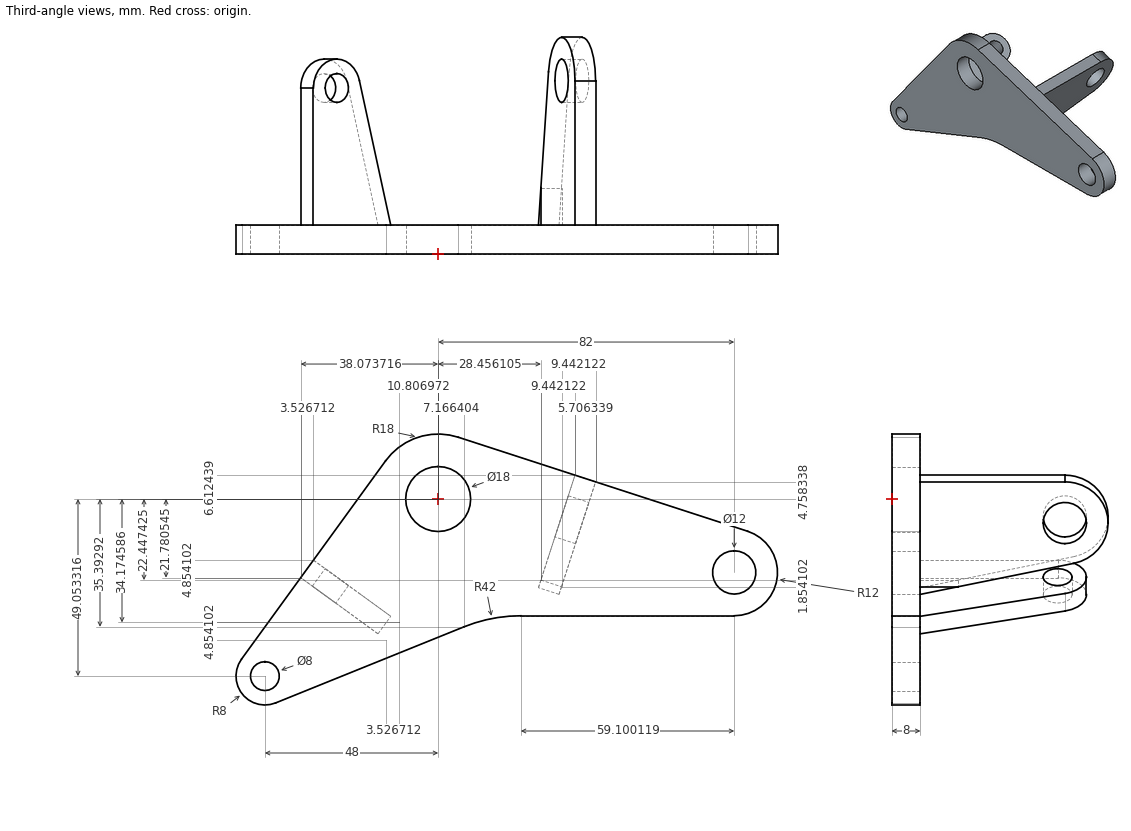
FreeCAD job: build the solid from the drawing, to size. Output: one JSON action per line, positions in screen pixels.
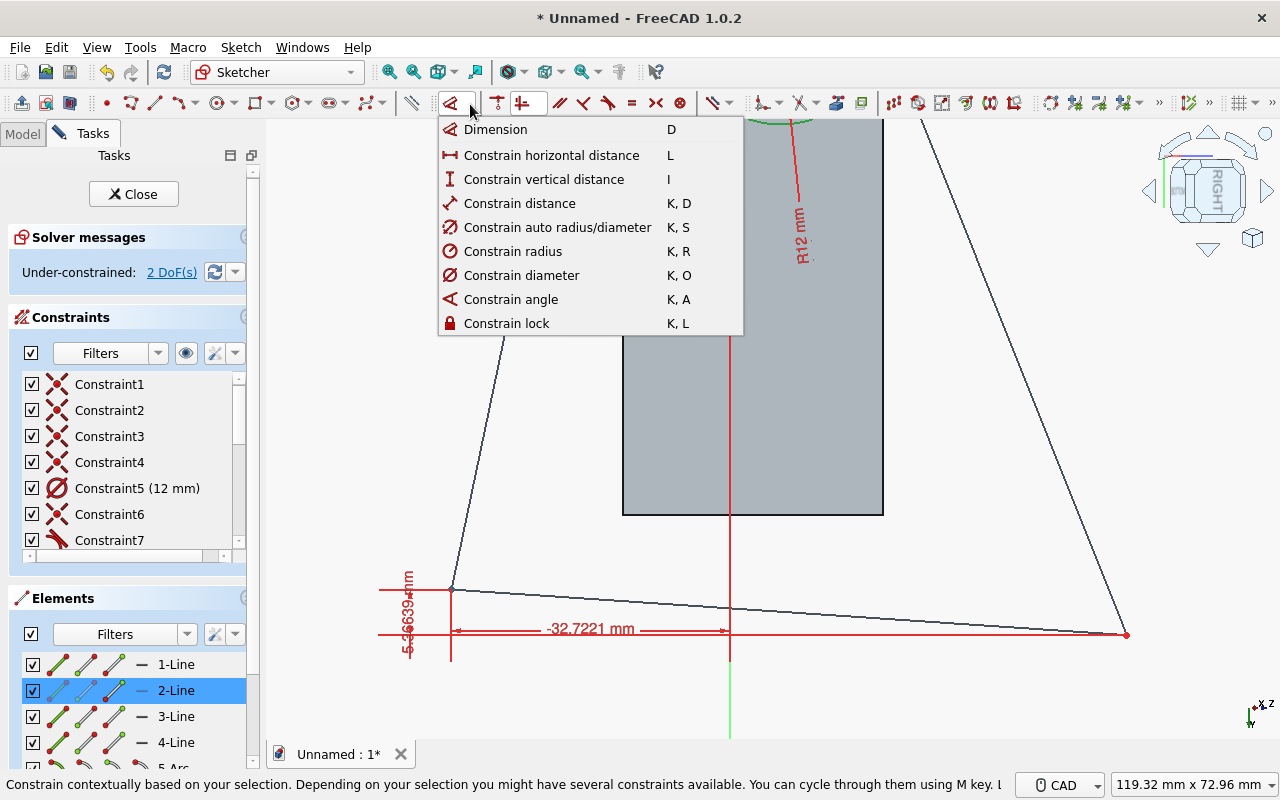
{"action": "left_click", "coordinate": [591, 179]}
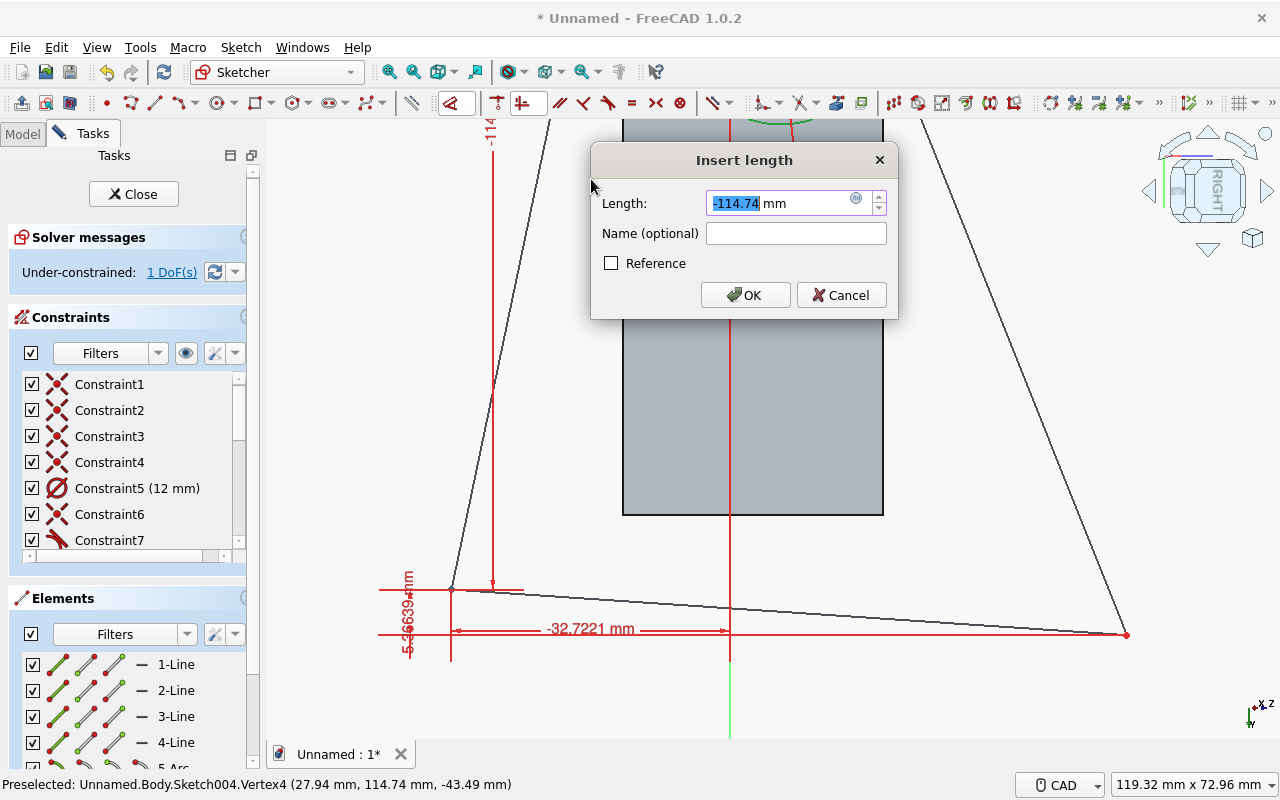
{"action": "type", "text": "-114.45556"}
{"action": "key", "text": "Return"}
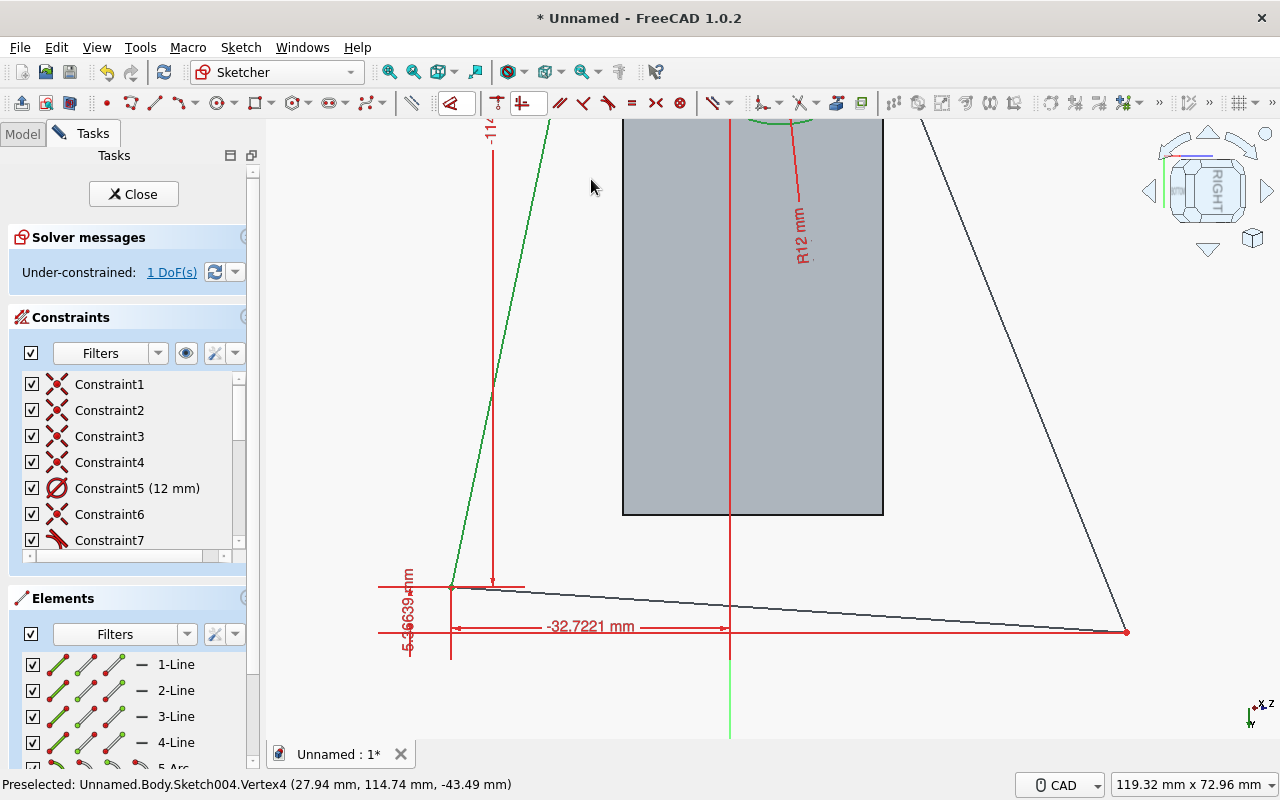
{"action": "scroll", "coordinate": [655, 607], "scroll_direction": "down", "scroll_amount": 5}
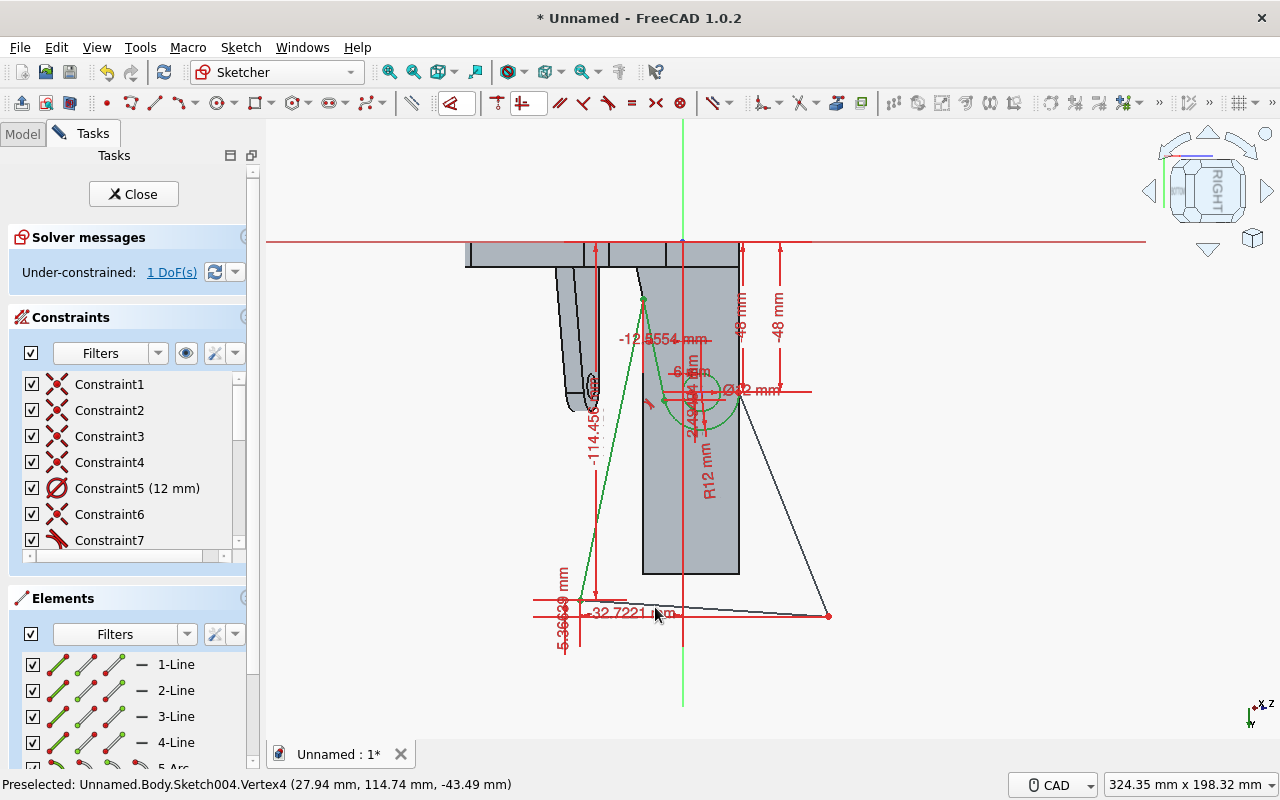
{"action": "left_click", "coordinate": [829, 617]}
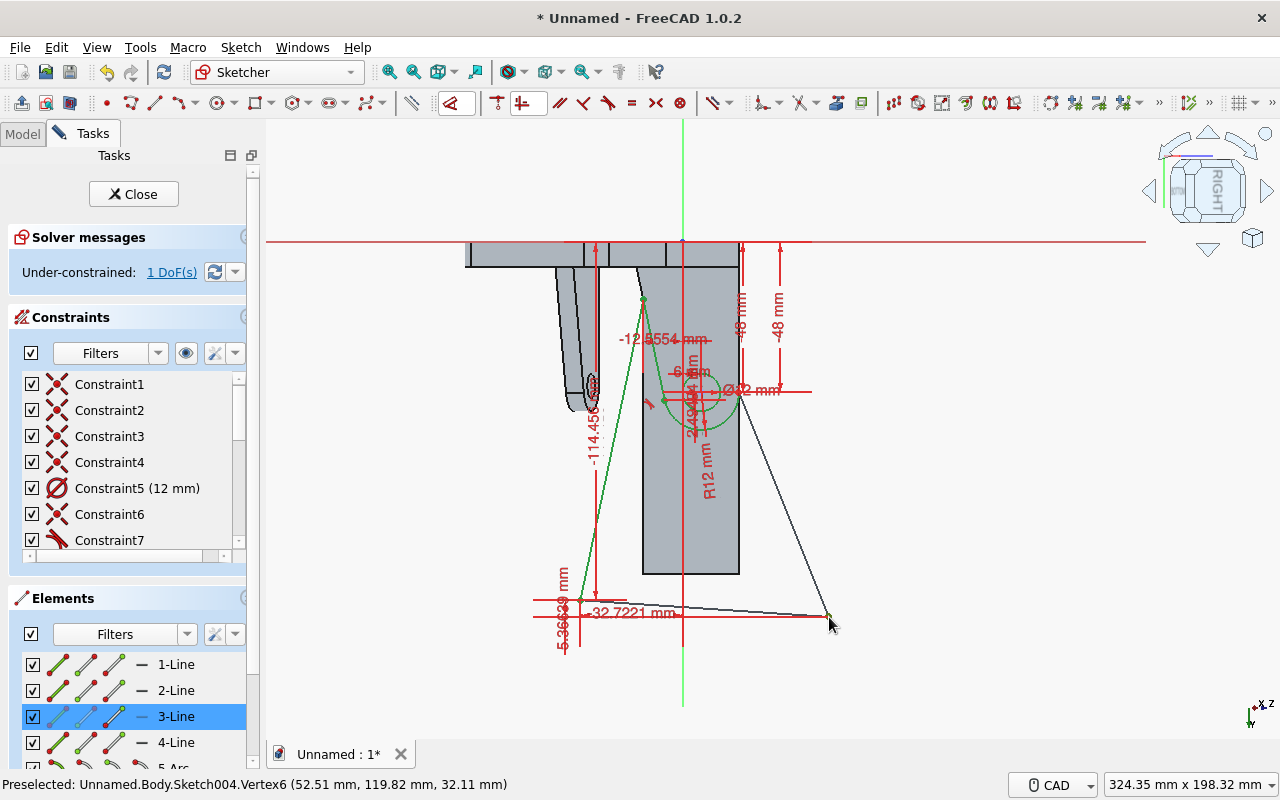
{"action": "key", "text": "l"}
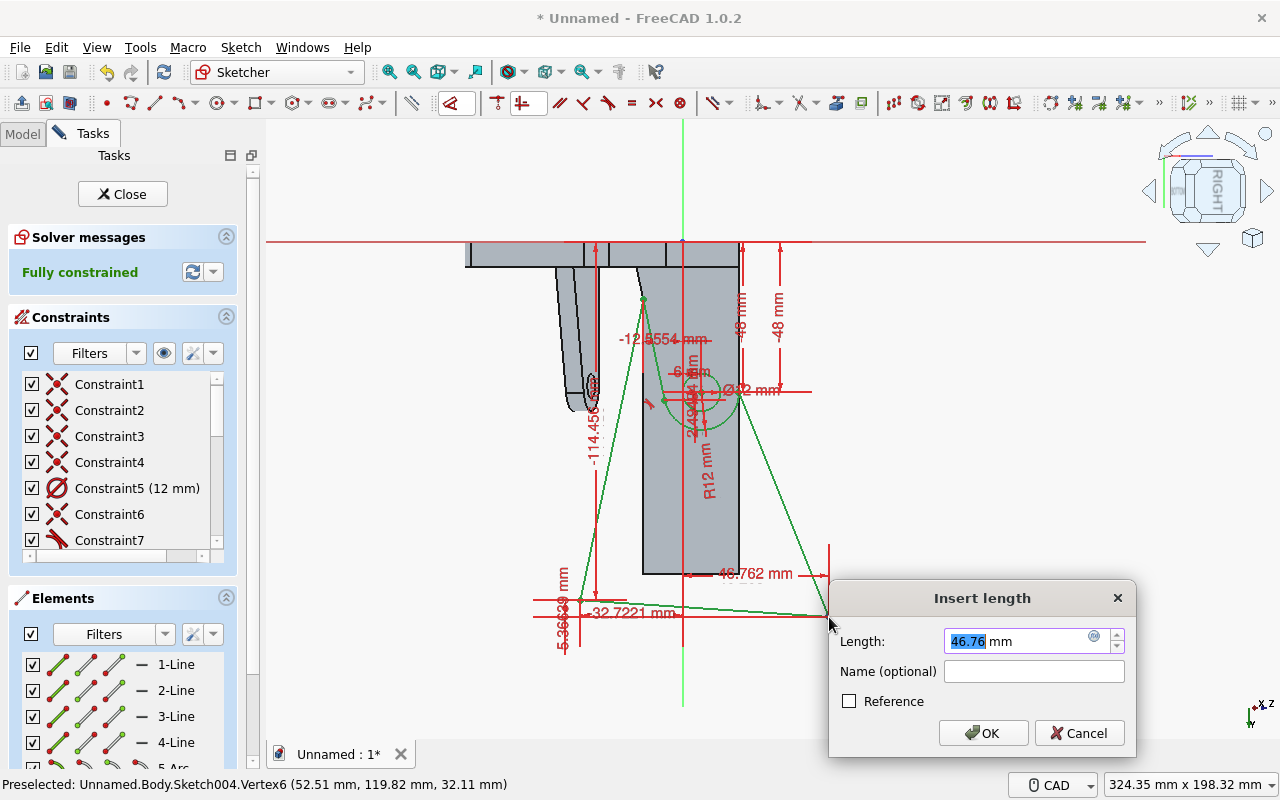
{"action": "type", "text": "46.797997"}
{"action": "key", "text": "Return"}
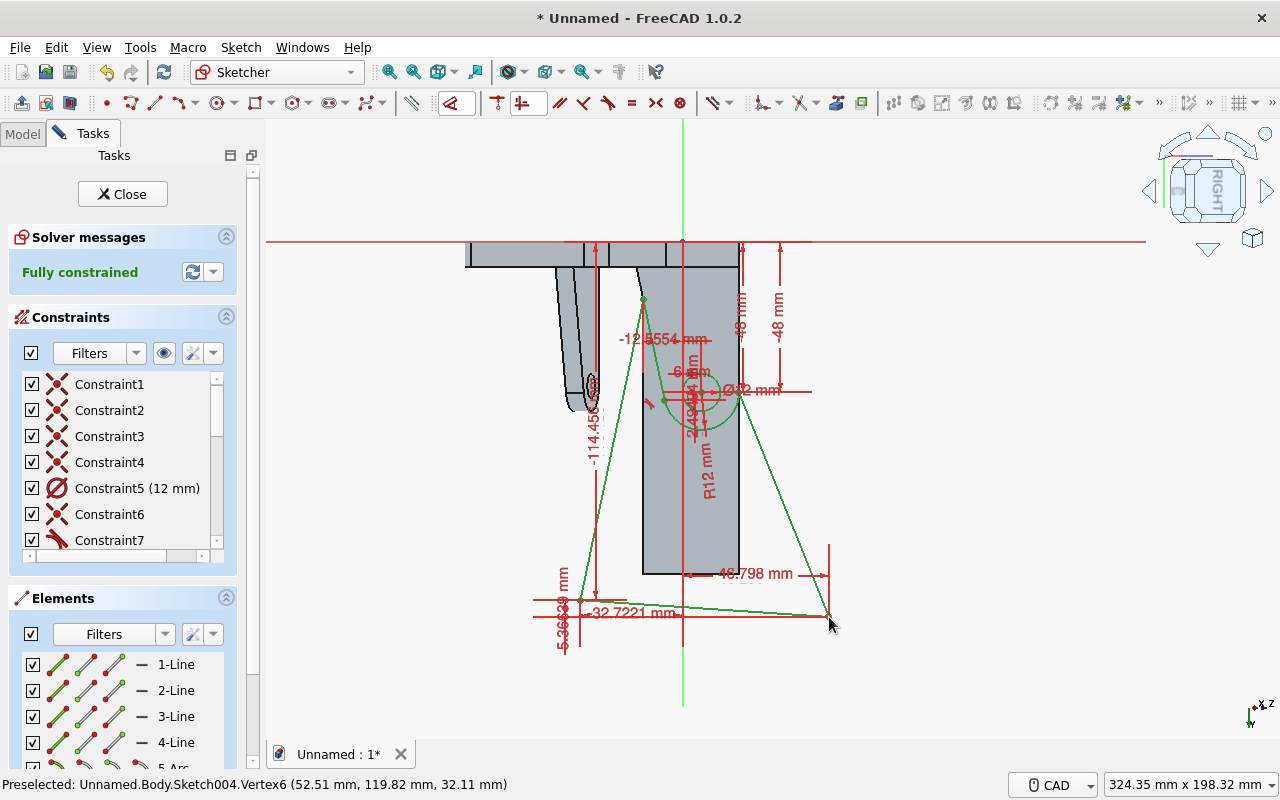
{"action": "left_click", "coordinate": [123, 194]}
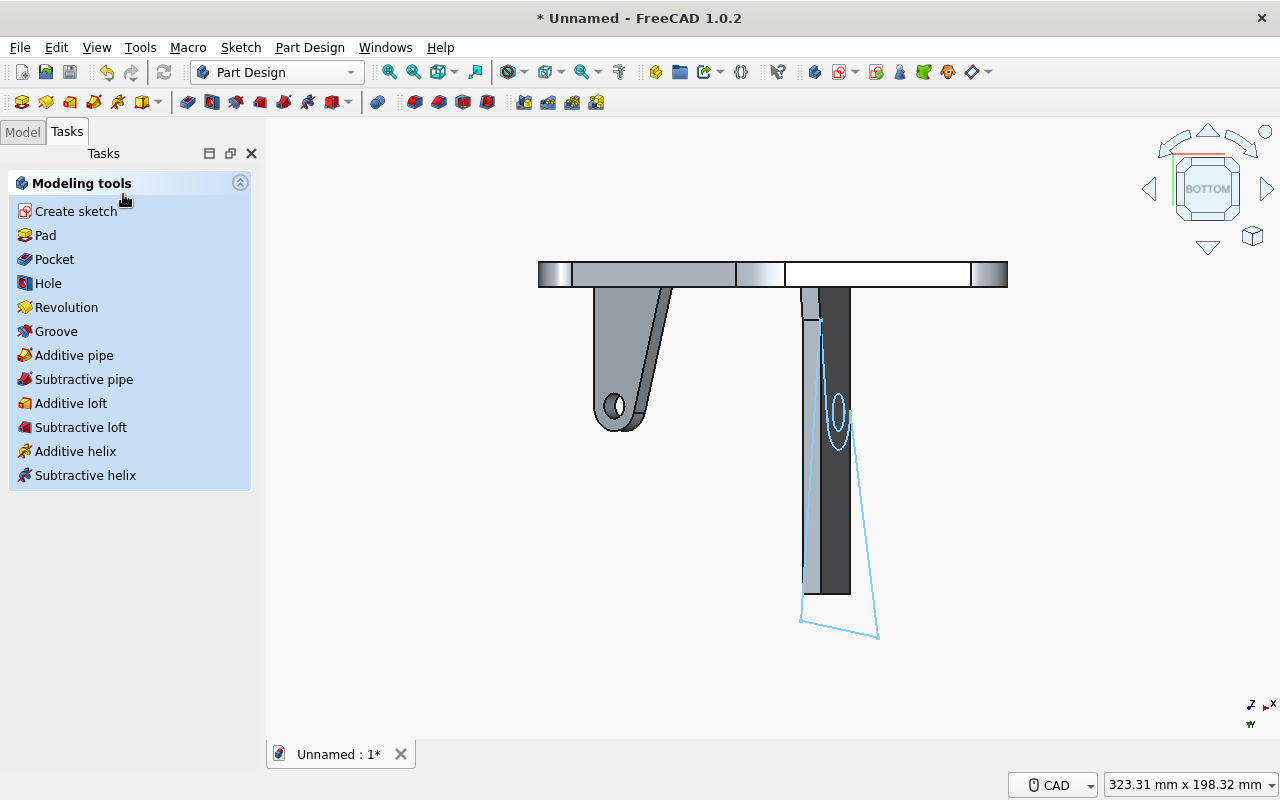
{"action": "left_click", "coordinate": [188, 102]}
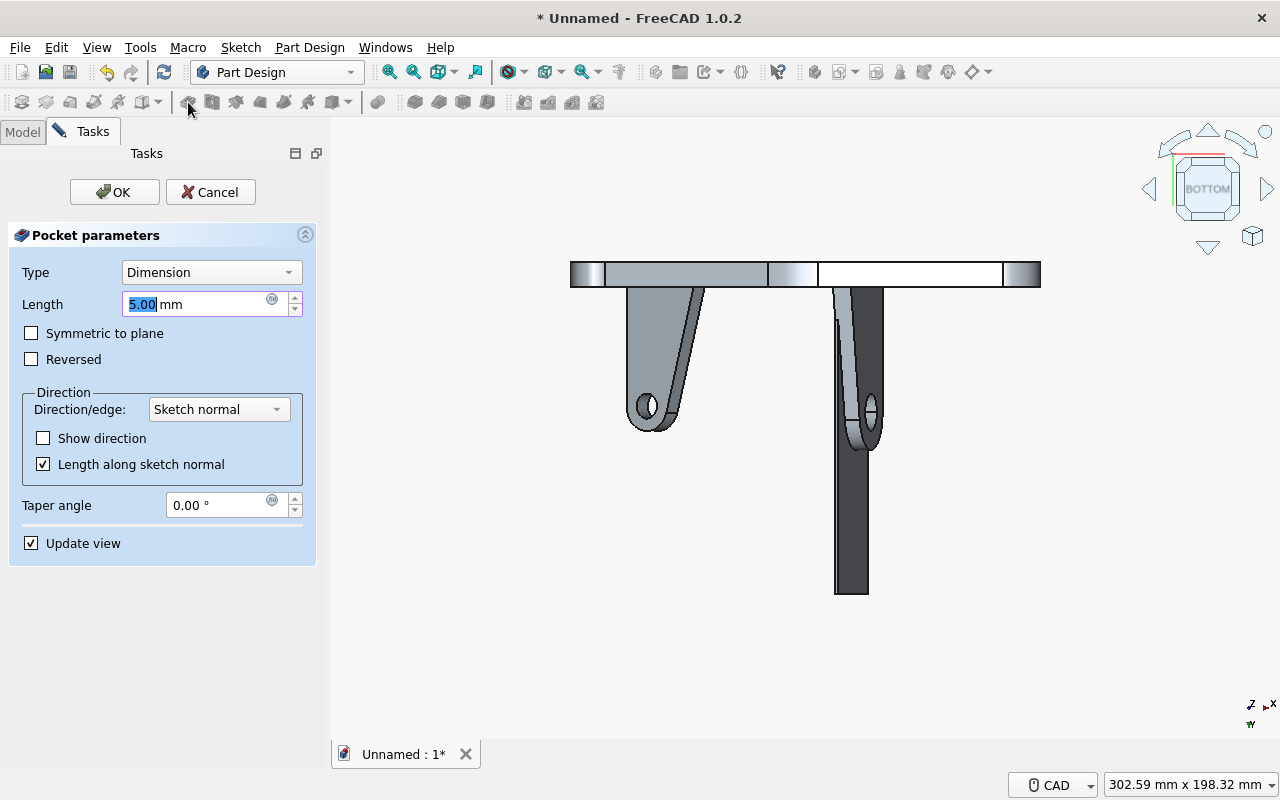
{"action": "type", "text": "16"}
{"action": "key", "text": "Tab"}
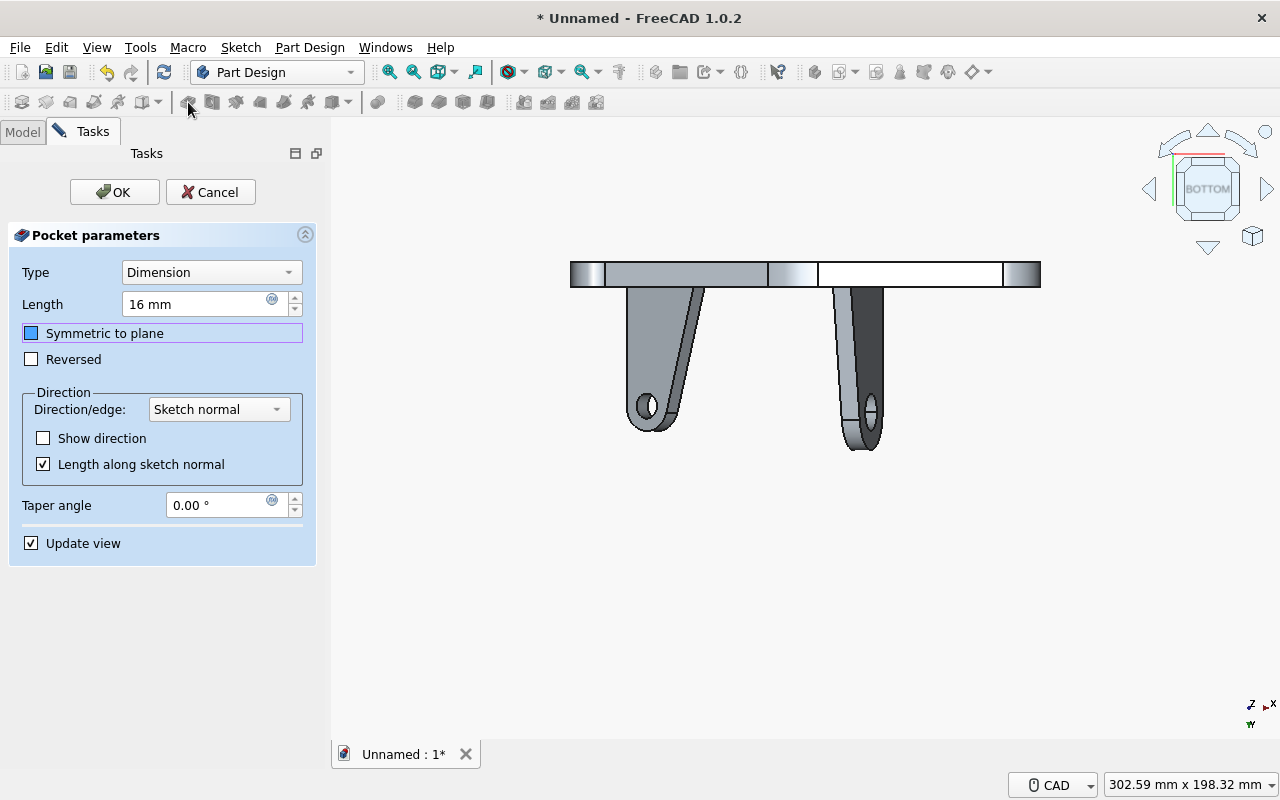
{"action": "left_click", "coordinate": [115, 192]}